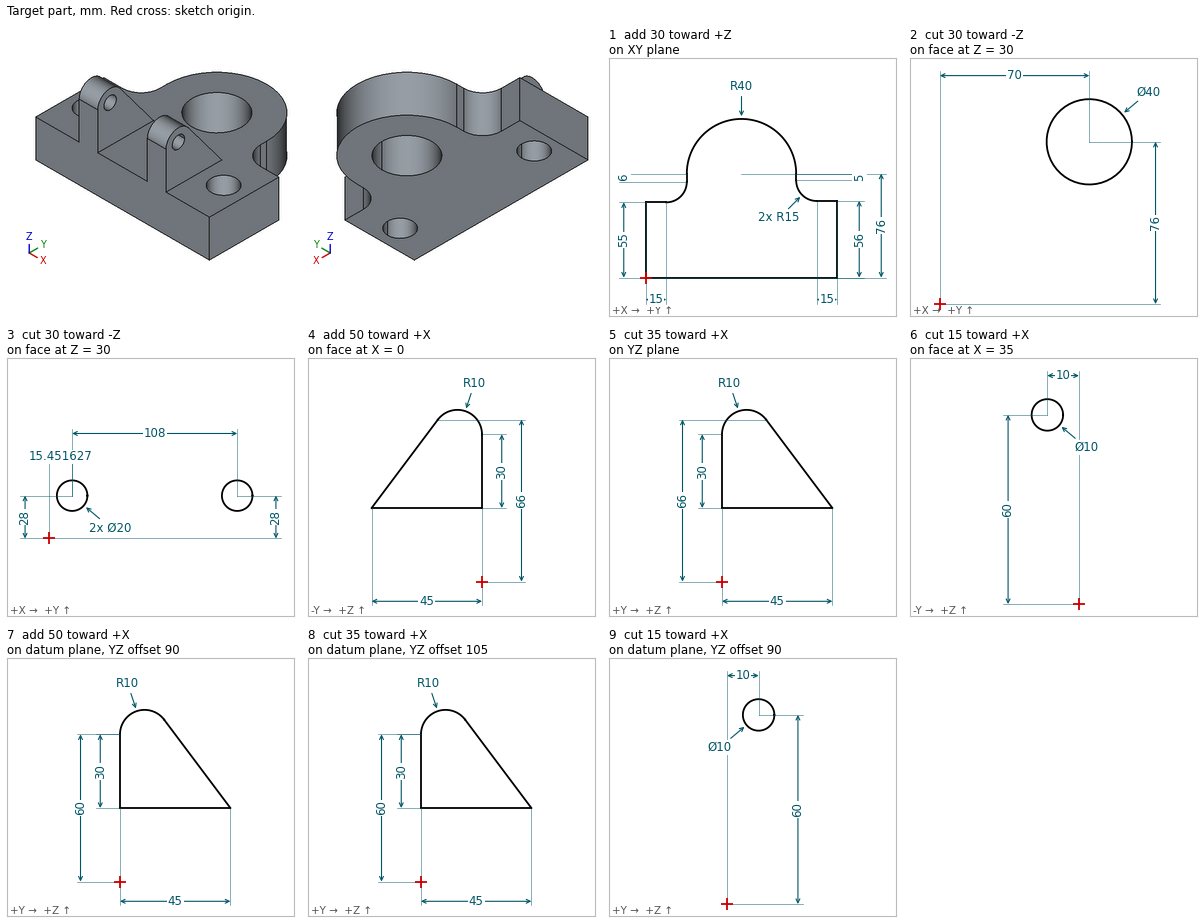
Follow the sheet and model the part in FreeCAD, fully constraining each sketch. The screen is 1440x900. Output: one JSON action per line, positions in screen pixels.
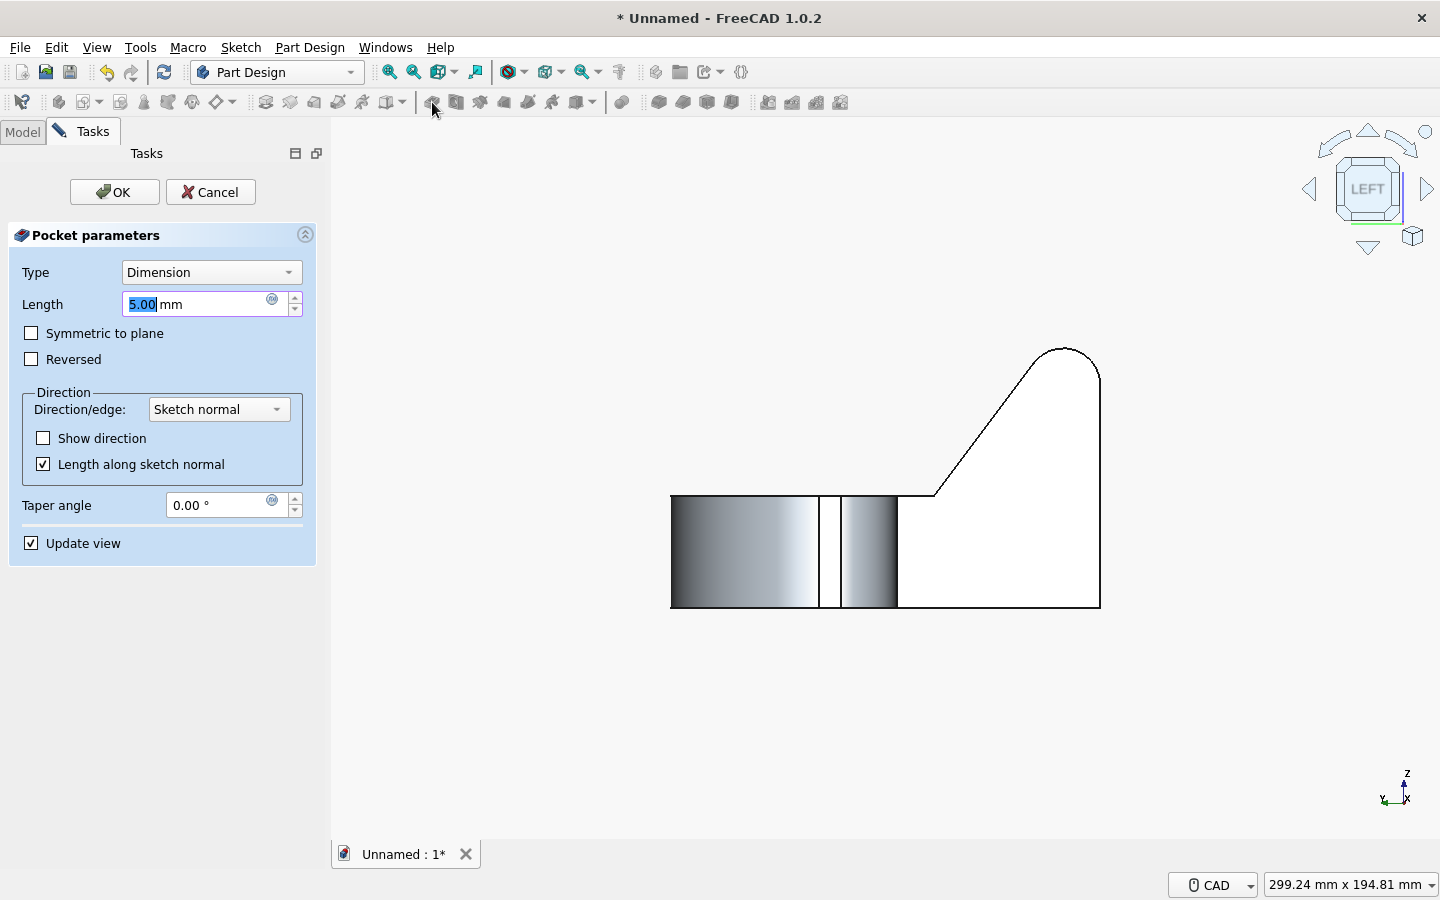
{"action": "type", "text": "35"}
{"action": "key", "text": "Tab"}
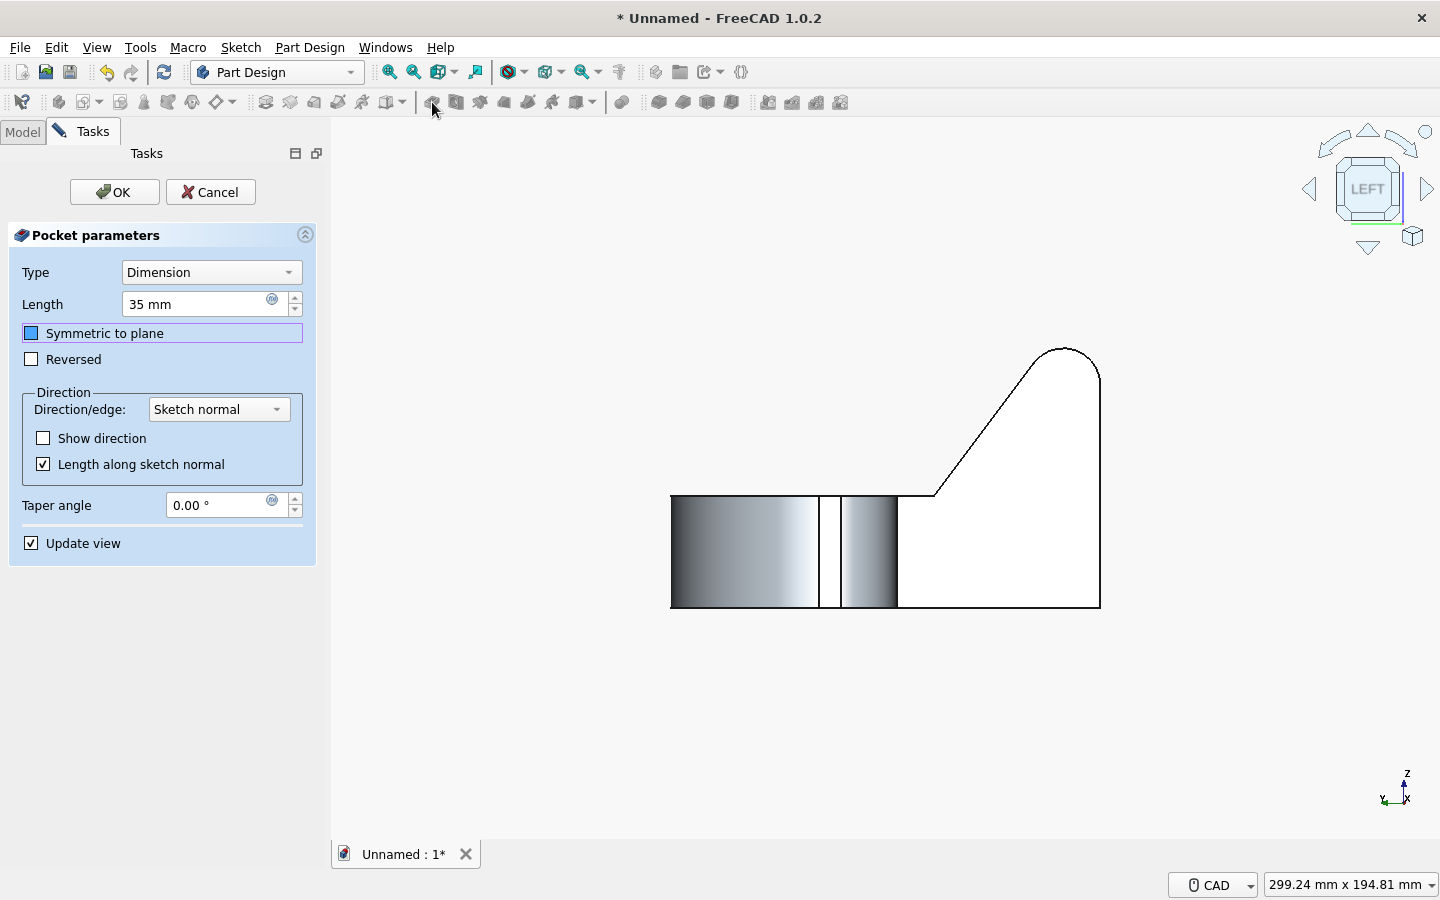
{"action": "left_click", "coordinate": [30, 359]}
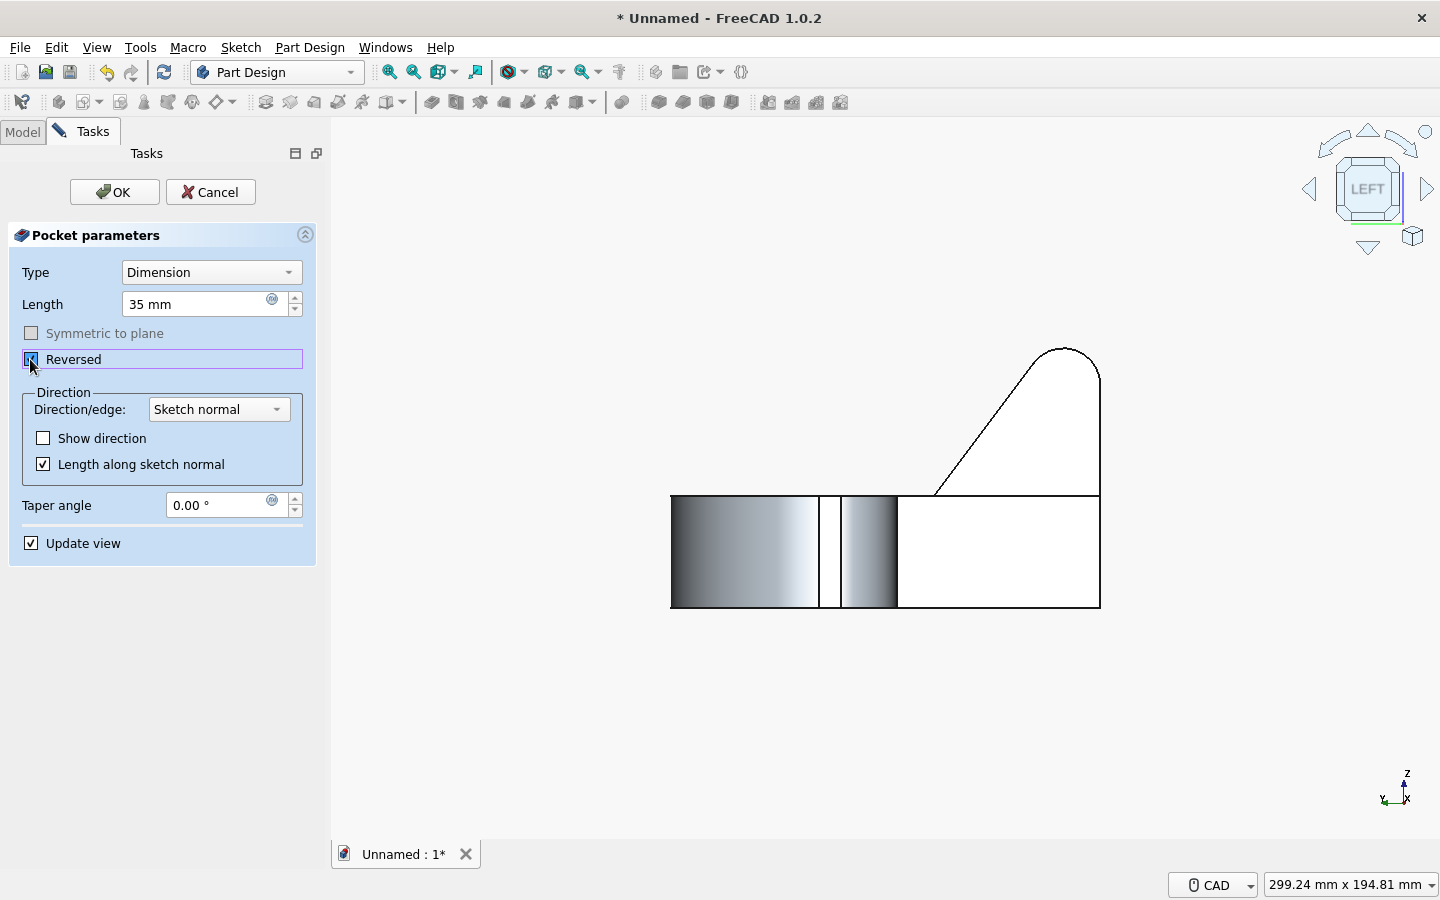
{"action": "left_click", "coordinate": [115, 192]}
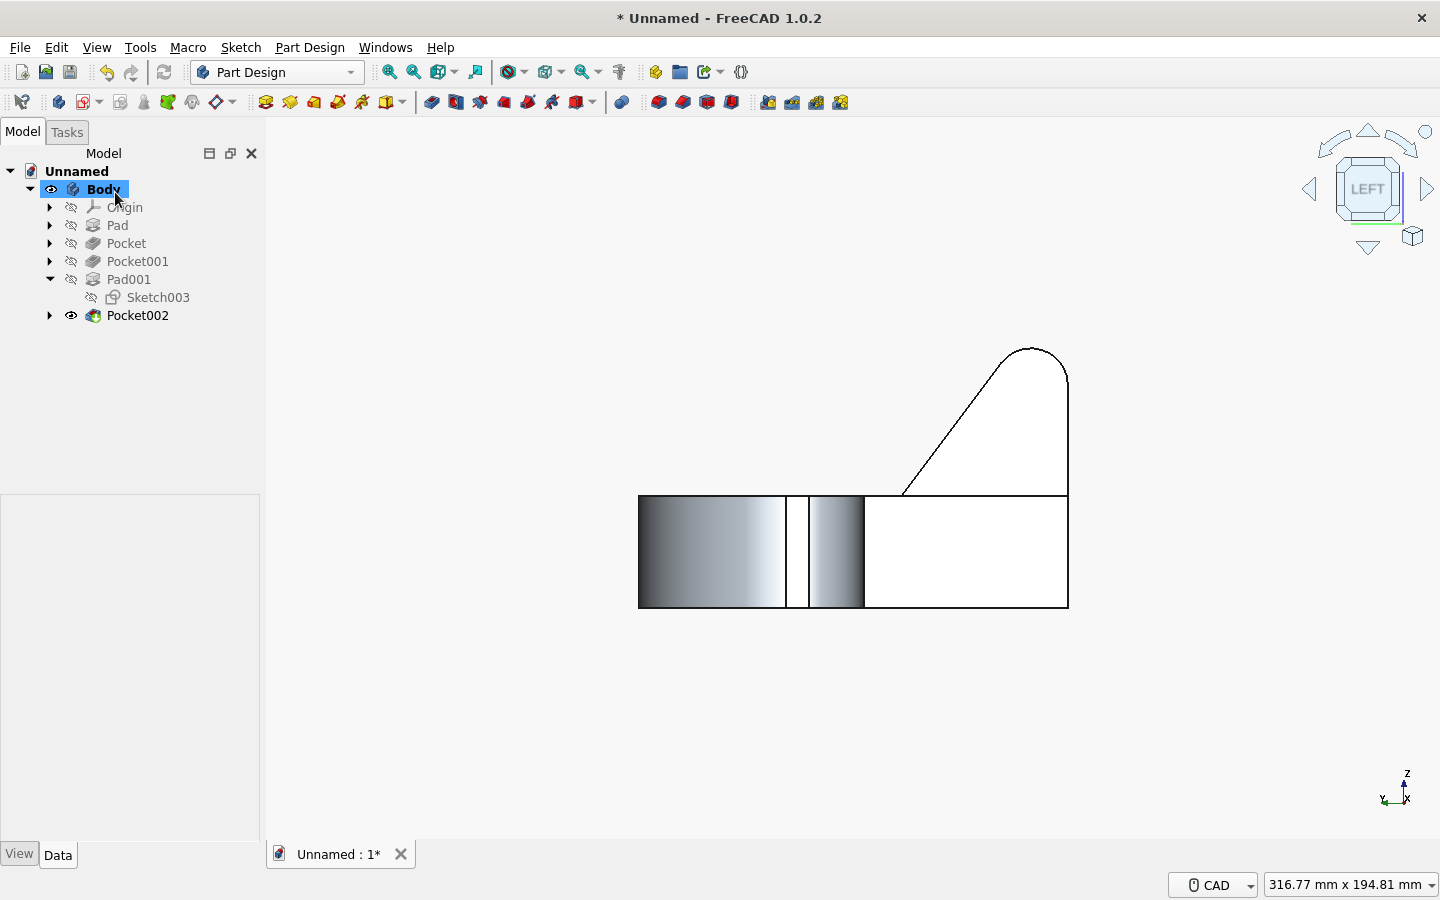
{"action": "key", "text": "v f"}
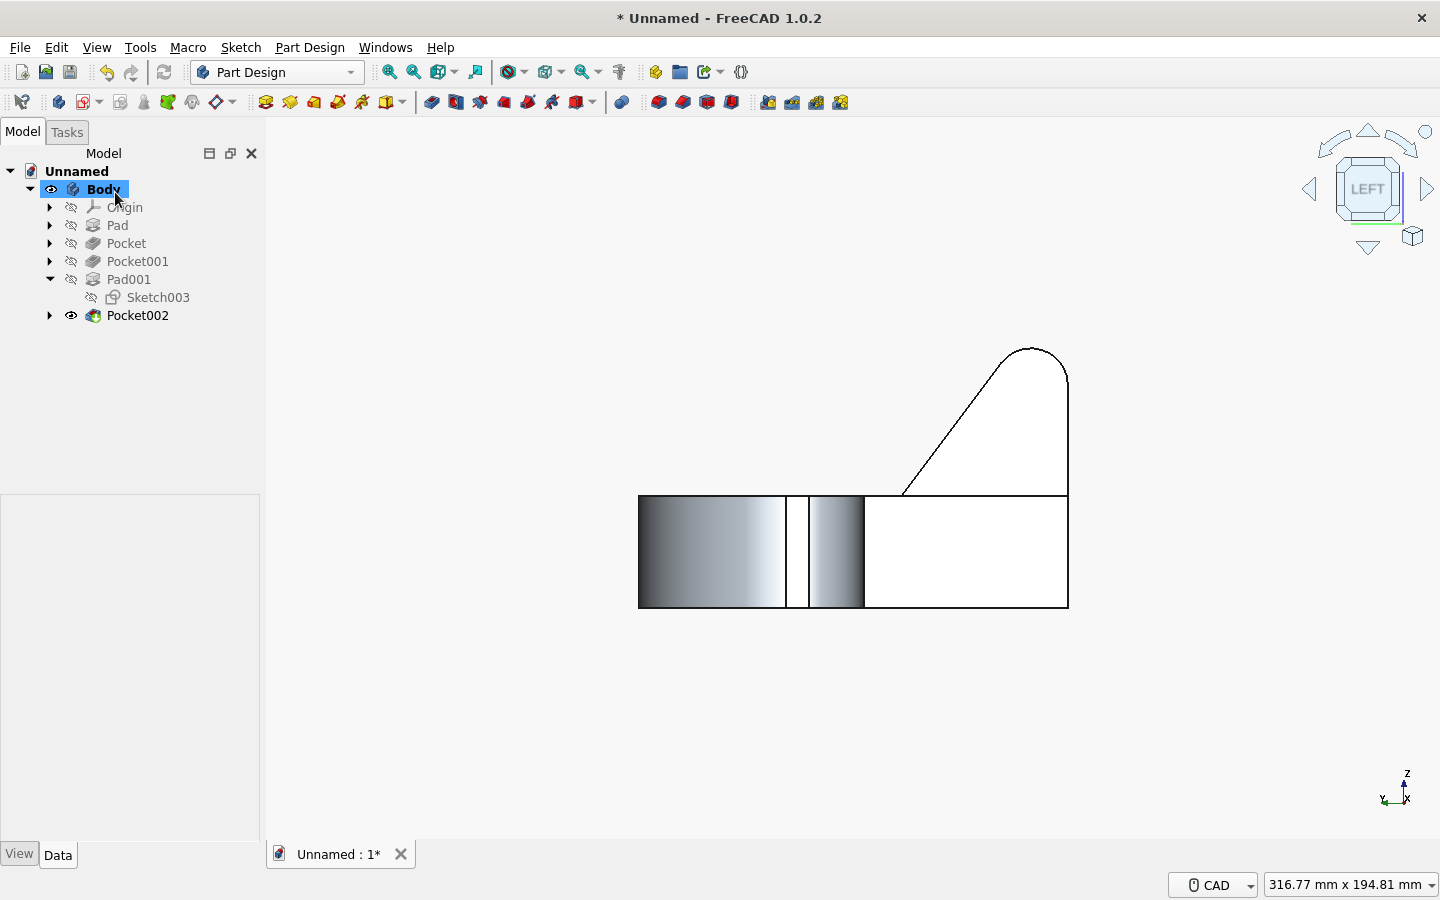
{"action": "left_click", "coordinate": [1008, 443]}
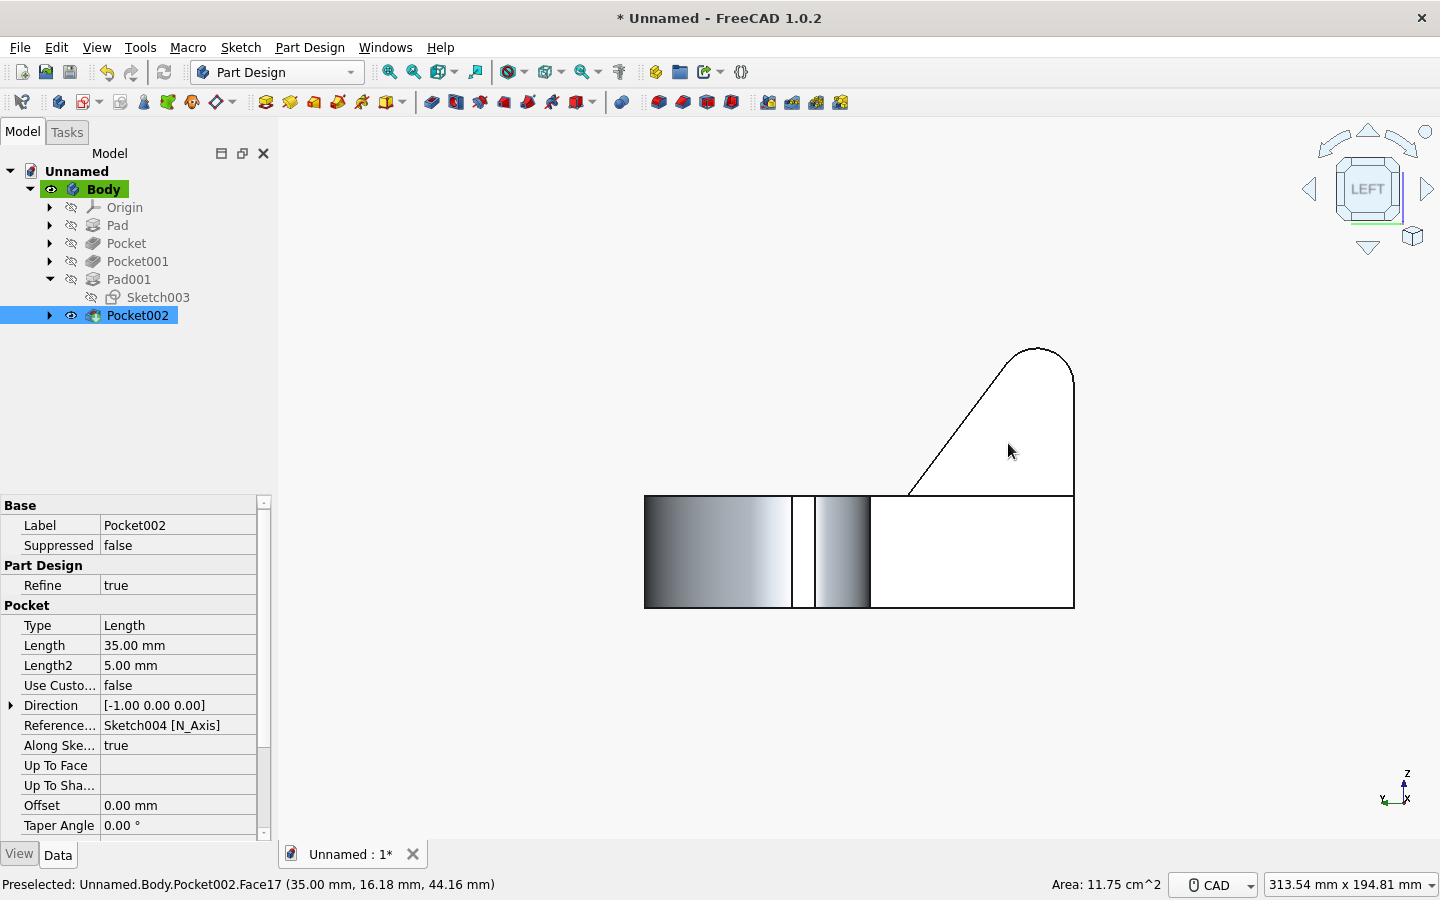
{"action": "left_click", "coordinate": [84, 102]}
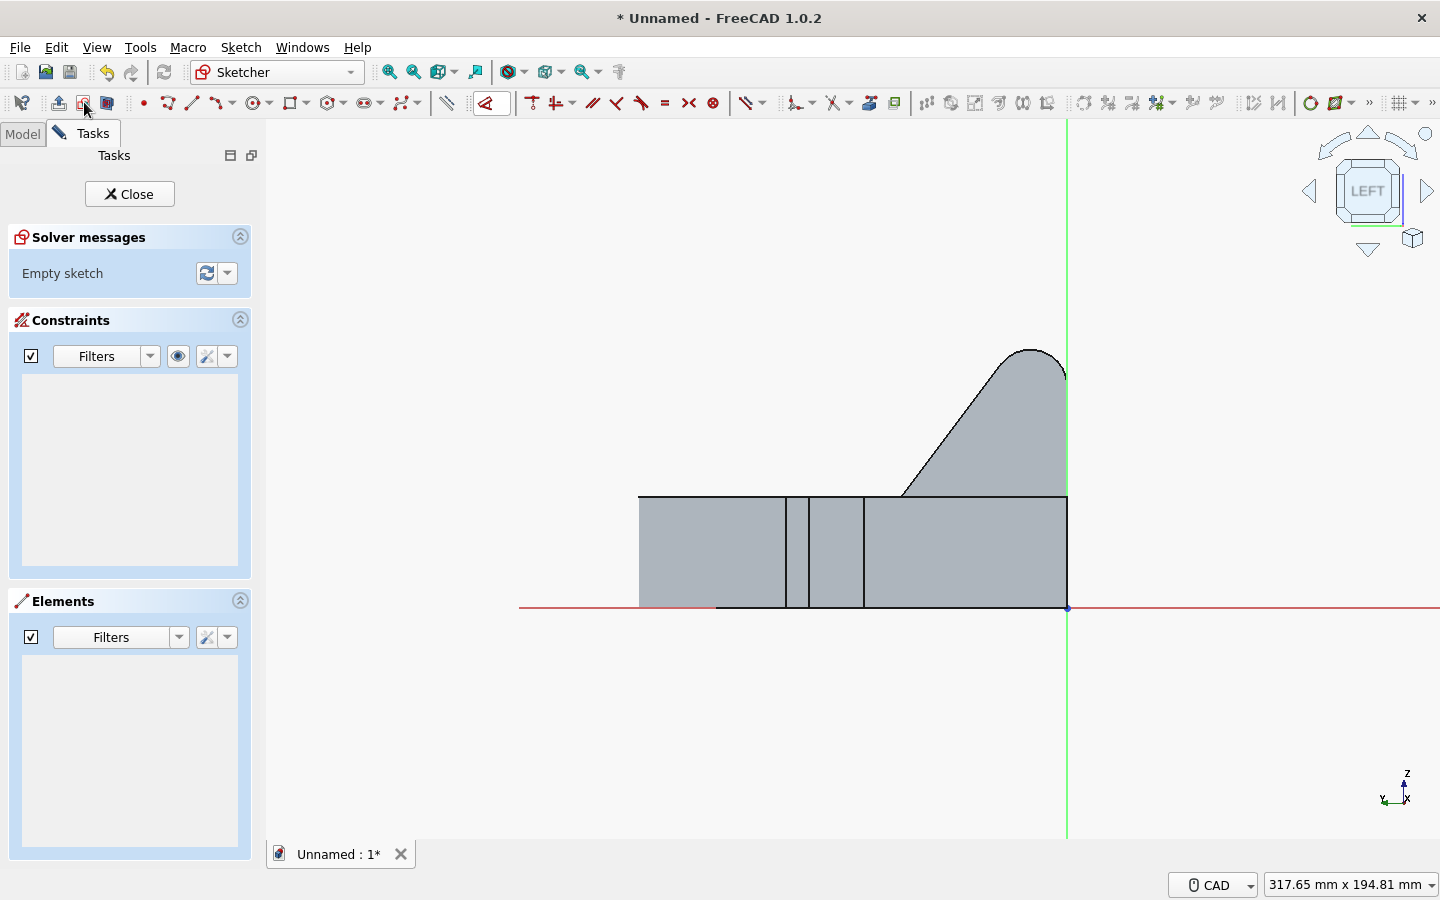
{"action": "scroll", "coordinate": [1050, 379], "scroll_direction": "up", "scroll_amount": 13}